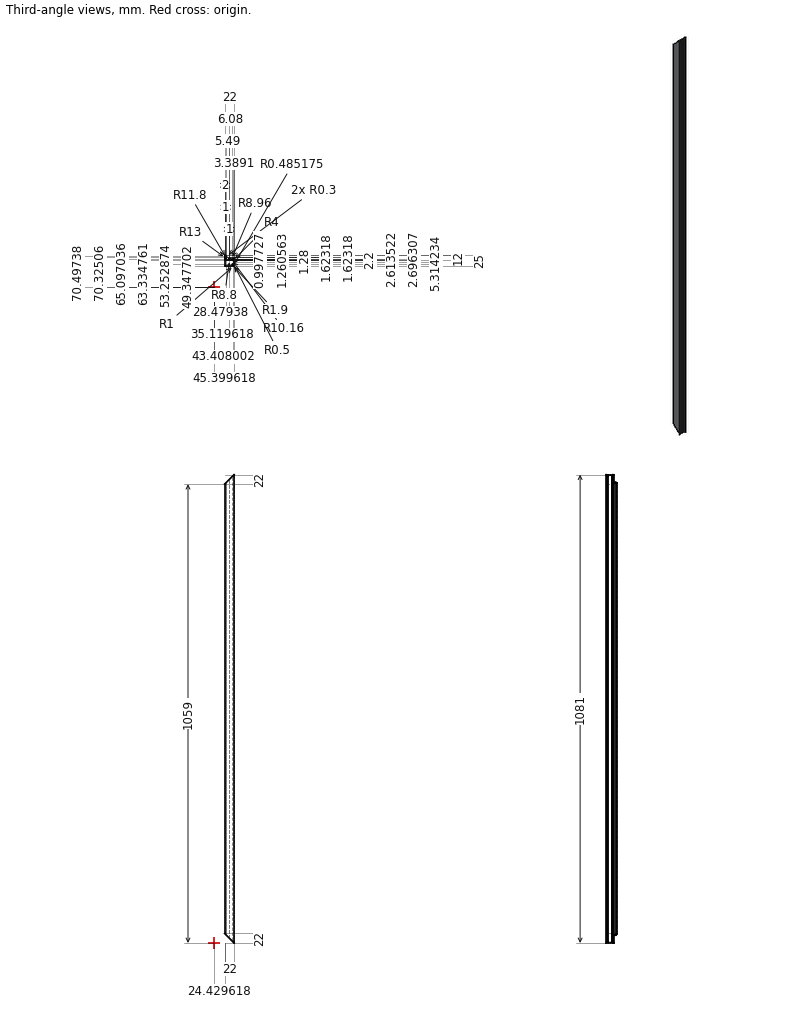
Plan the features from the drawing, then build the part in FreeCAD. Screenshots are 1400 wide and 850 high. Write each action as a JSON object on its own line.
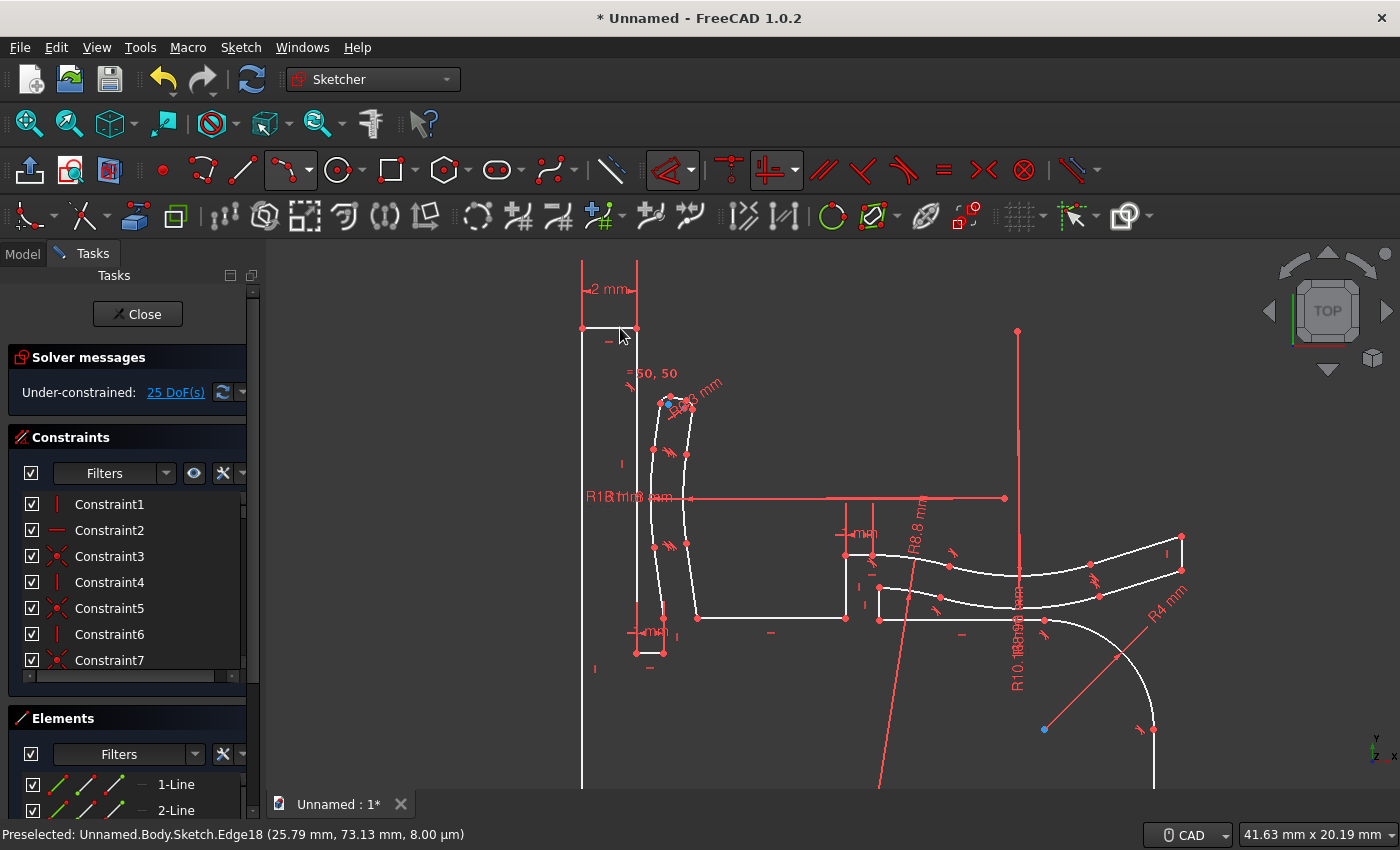
{"action": "left_click", "coordinate": [637, 556]}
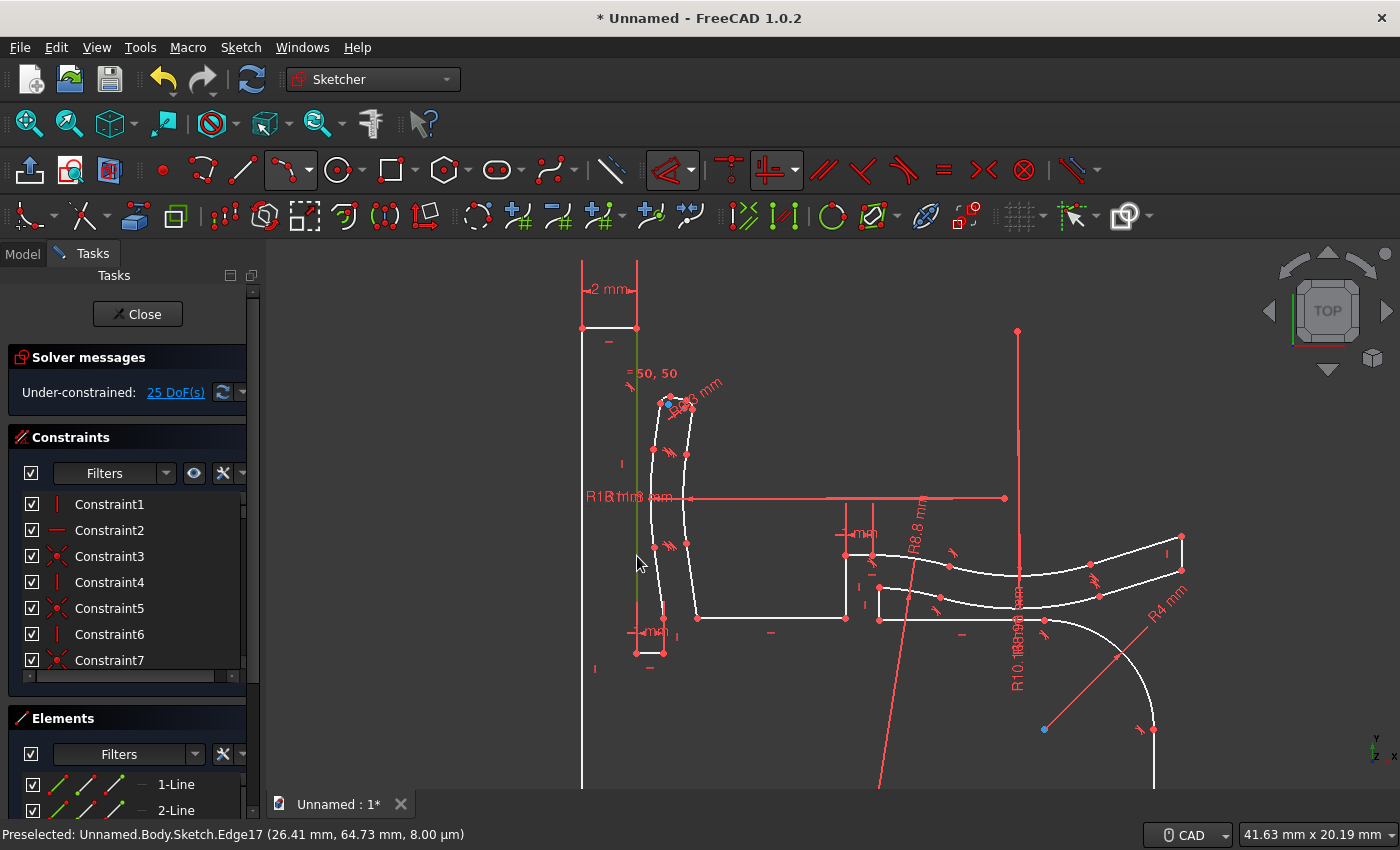
{"action": "left_click", "coordinate": [694, 170]}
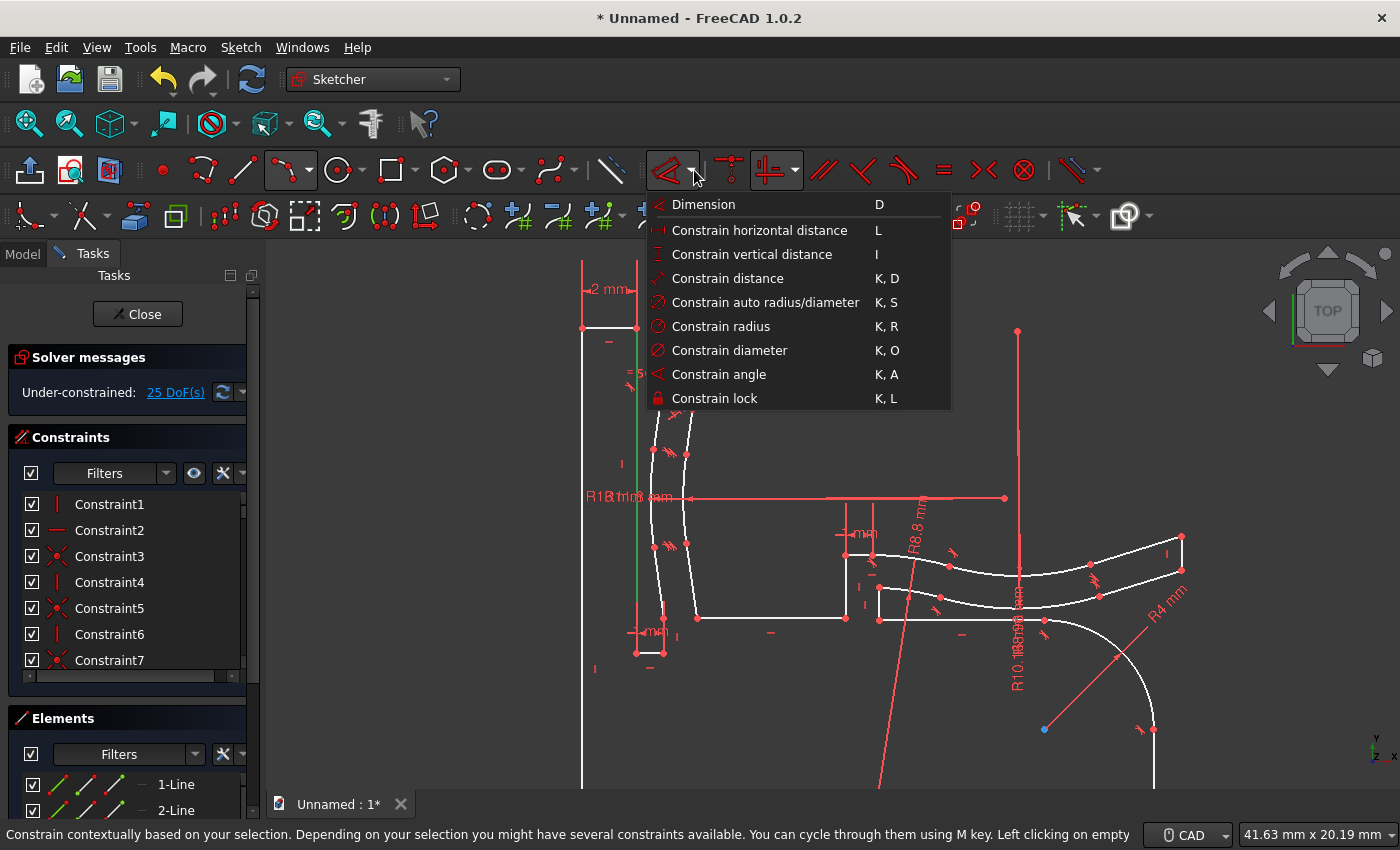
{"action": "left_click", "coordinate": [799, 254]}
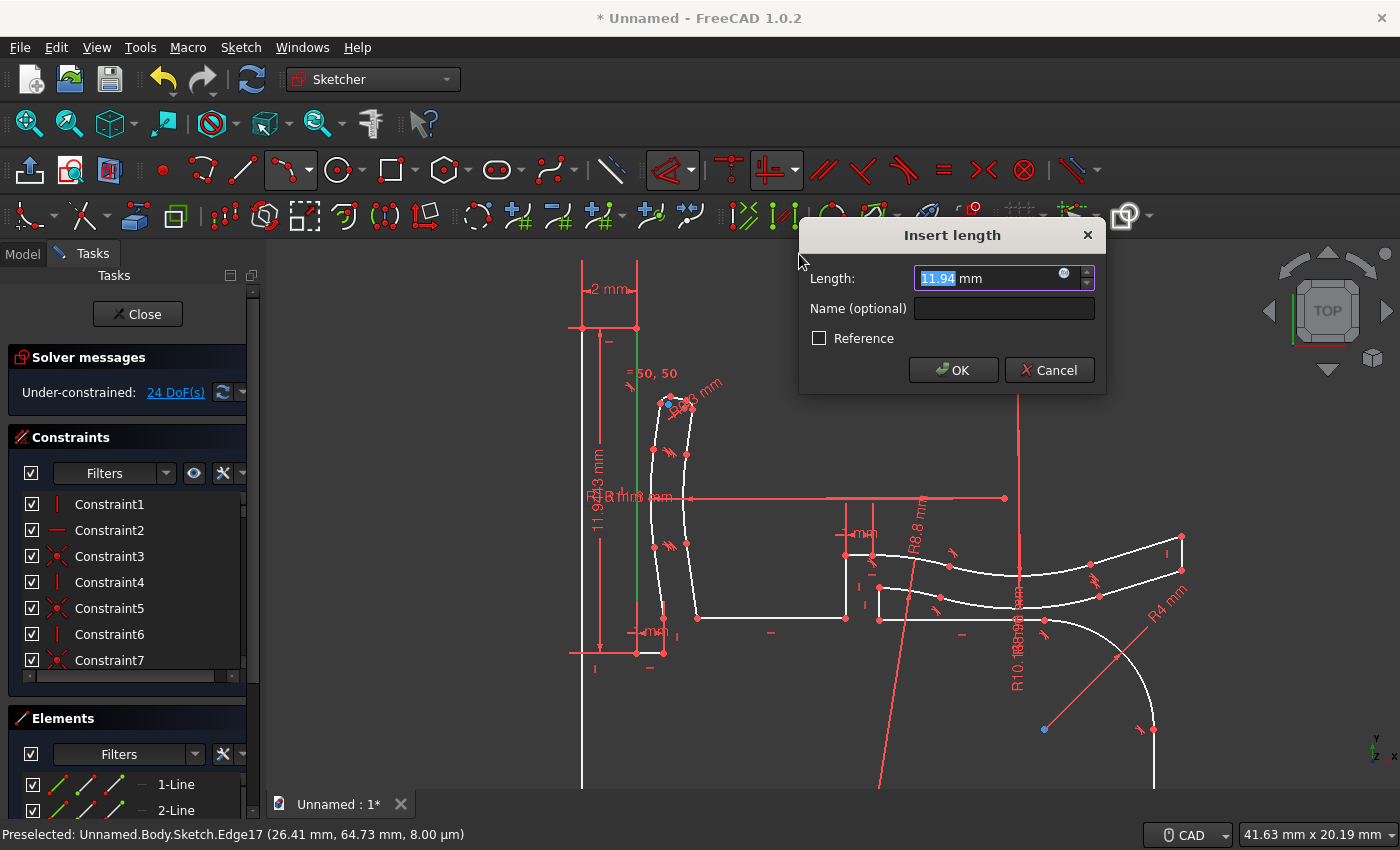
{"action": "type", "text": "12"}
{"action": "key", "text": "Return"}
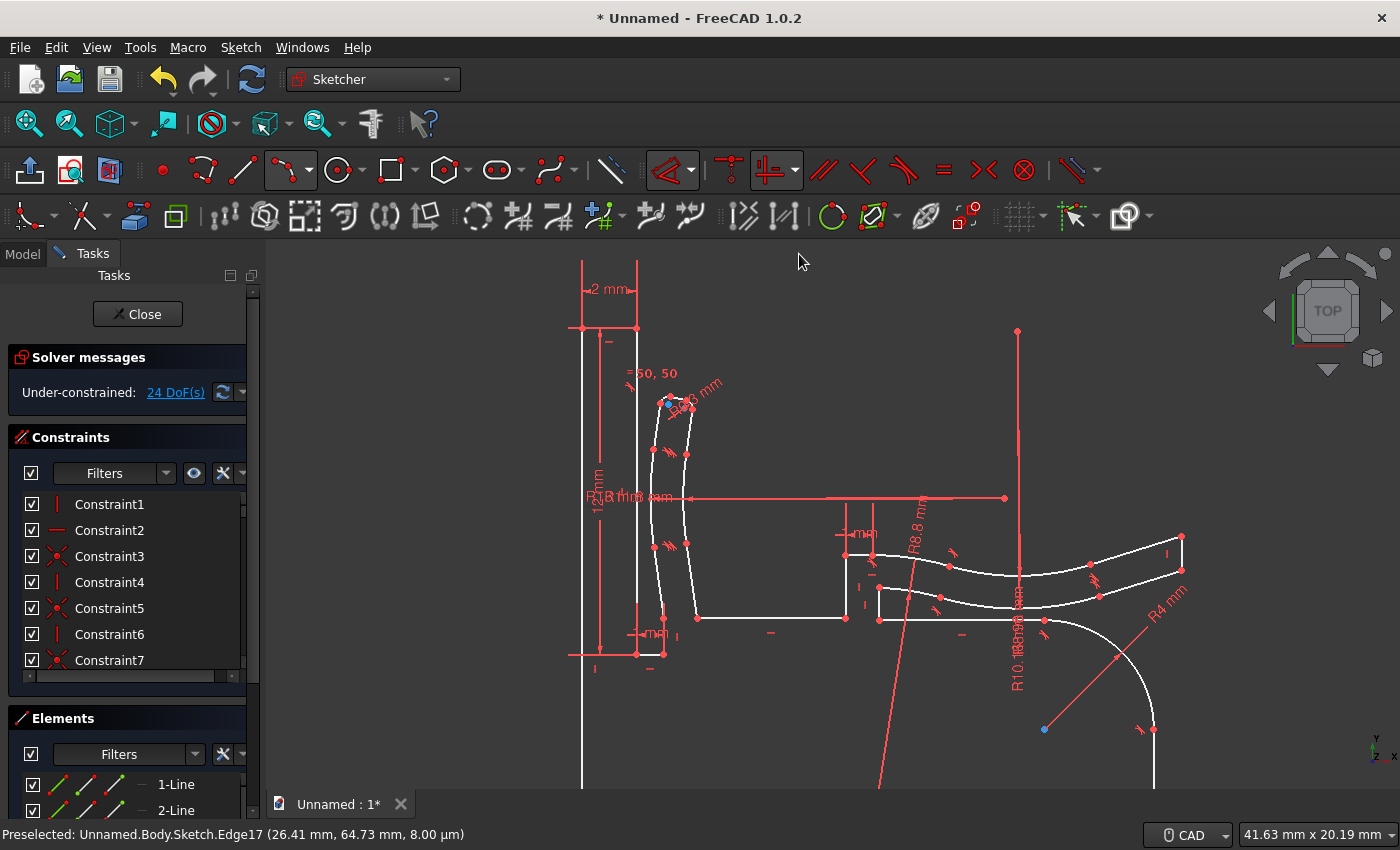
{"action": "left_click", "coordinate": [582, 533]}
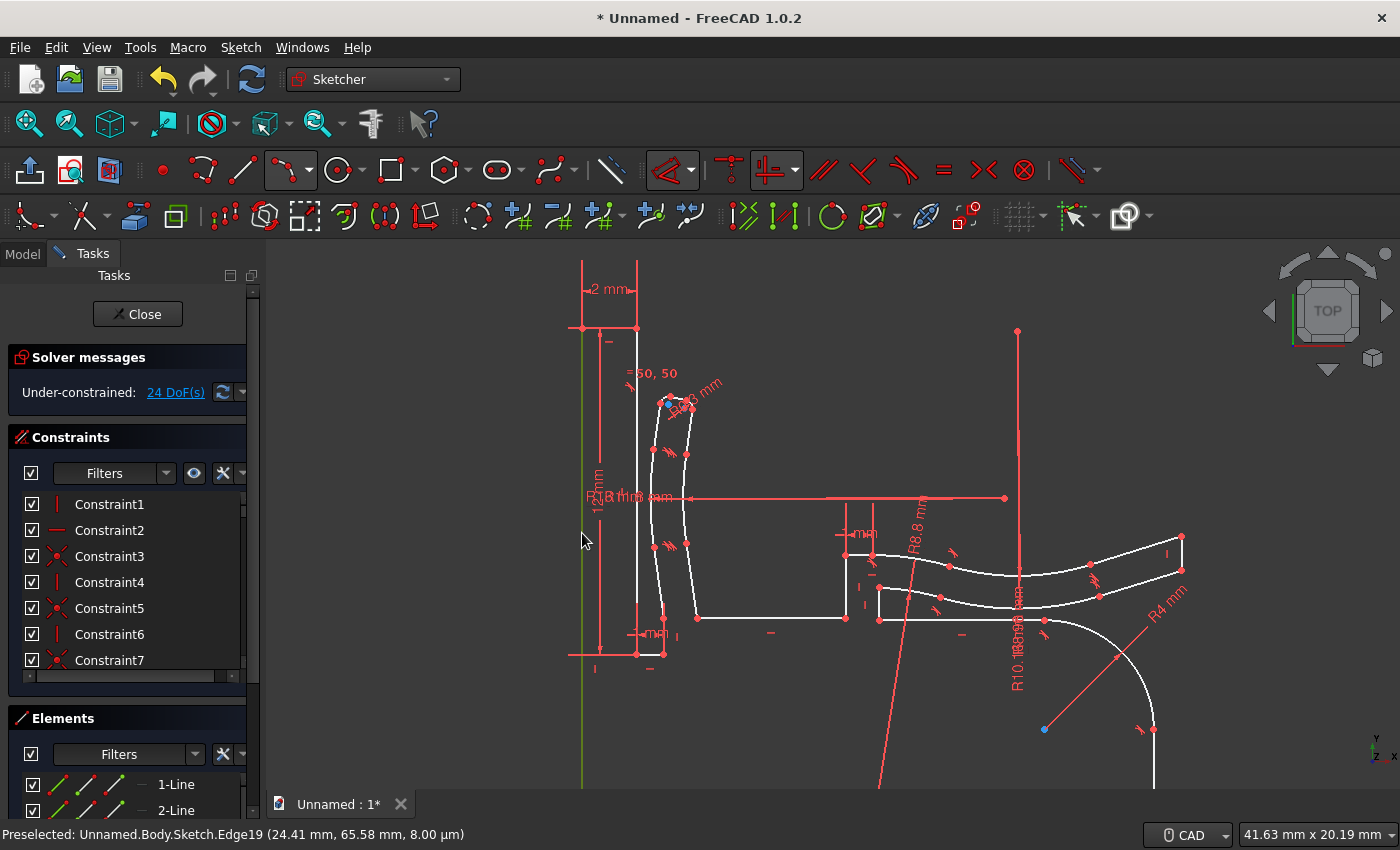
{"action": "left_click", "coordinate": [694, 170]}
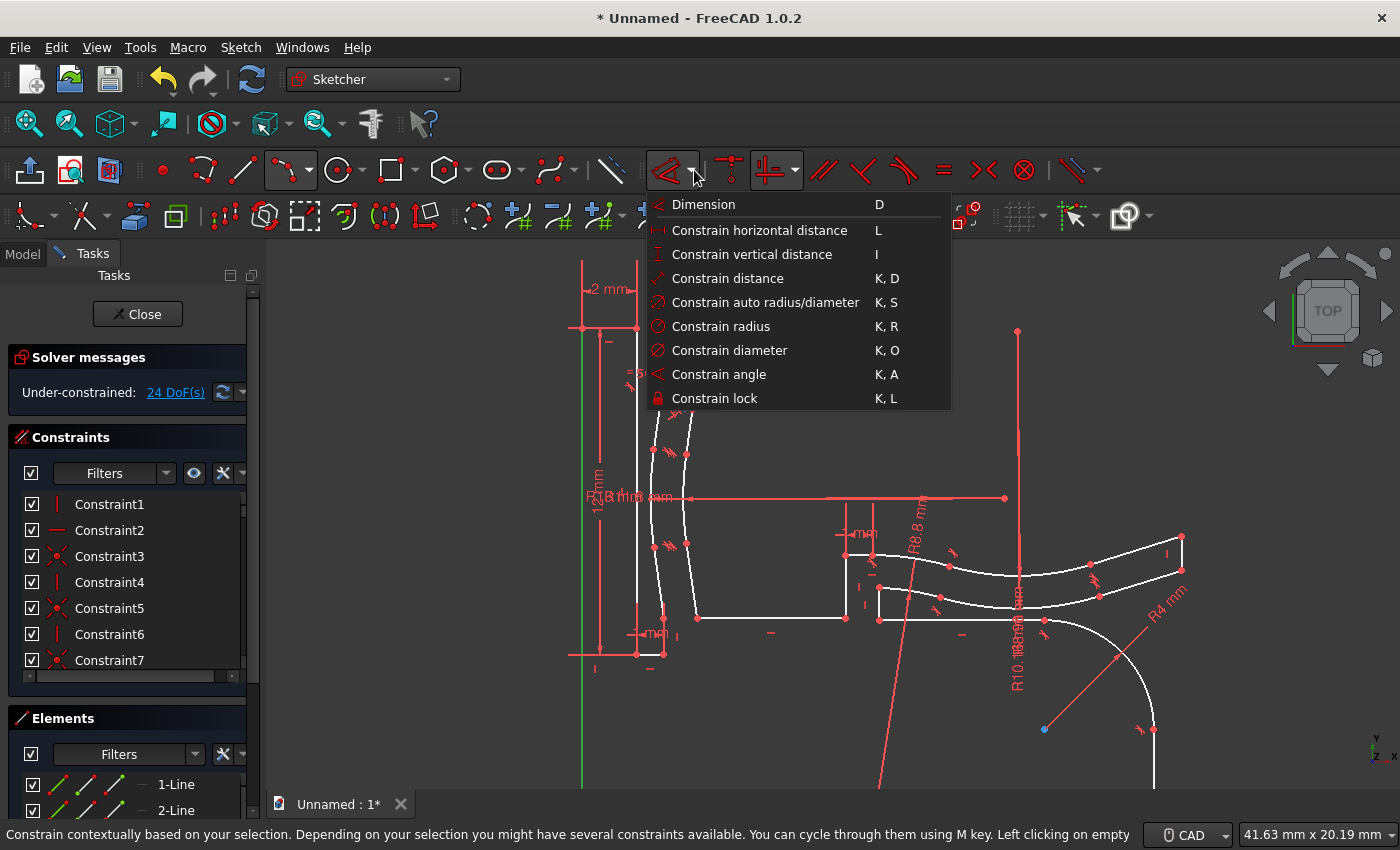
{"action": "left_click", "coordinate": [799, 254]}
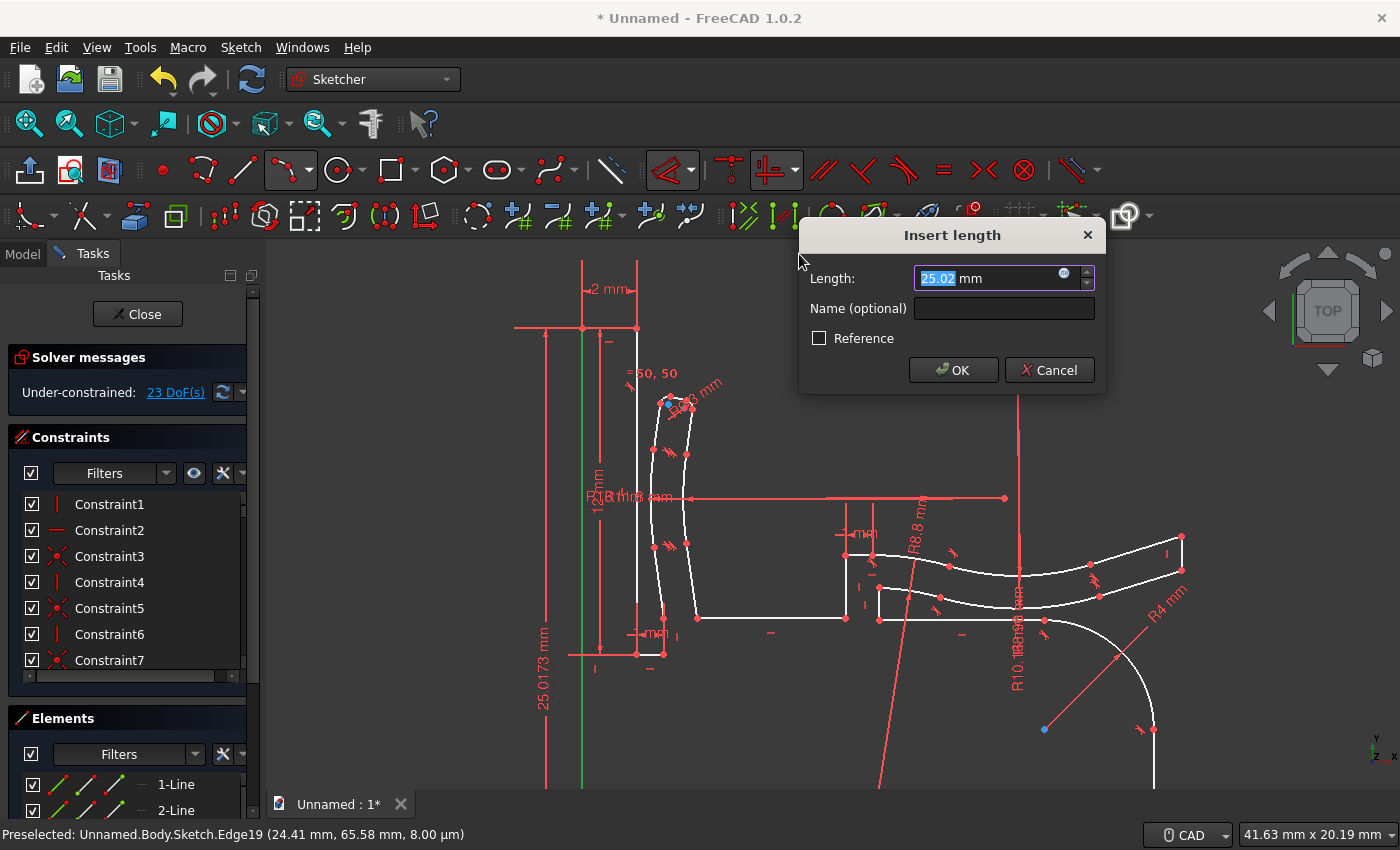
{"action": "type", "text": "25"}
{"action": "key", "text": "Return"}